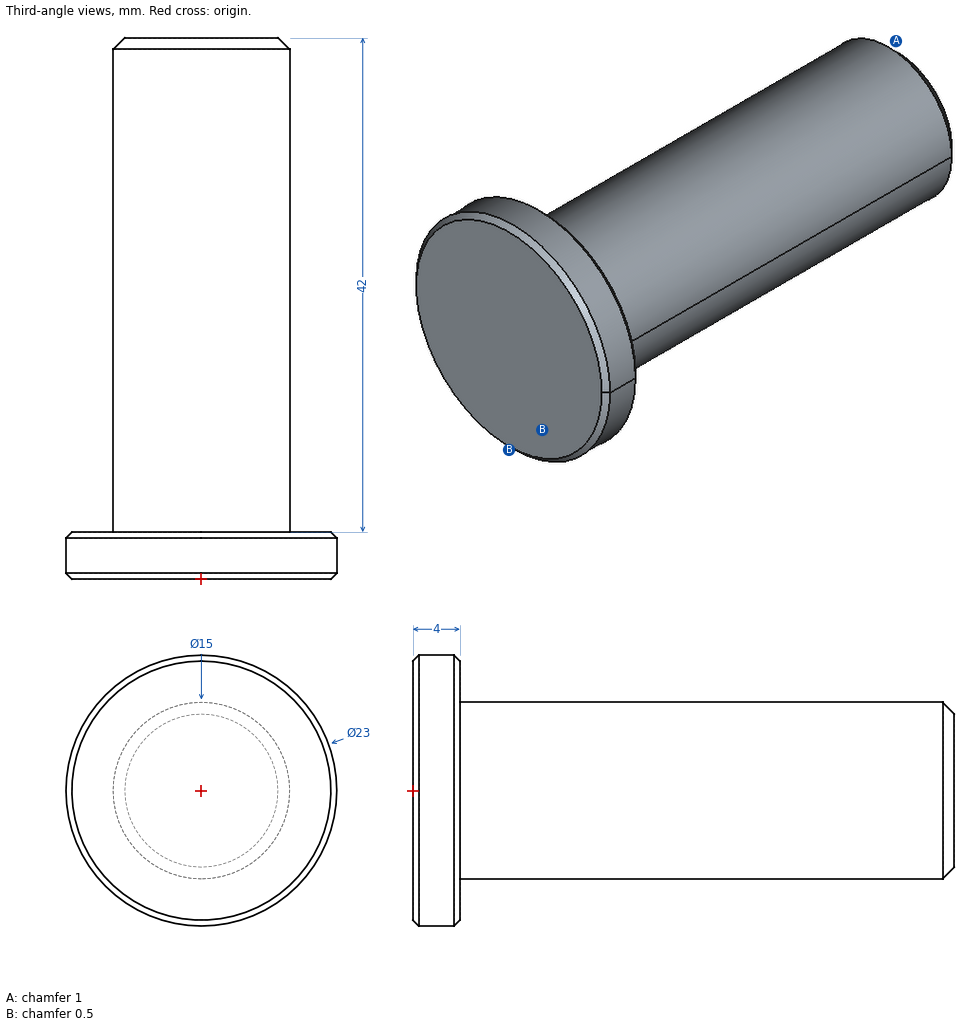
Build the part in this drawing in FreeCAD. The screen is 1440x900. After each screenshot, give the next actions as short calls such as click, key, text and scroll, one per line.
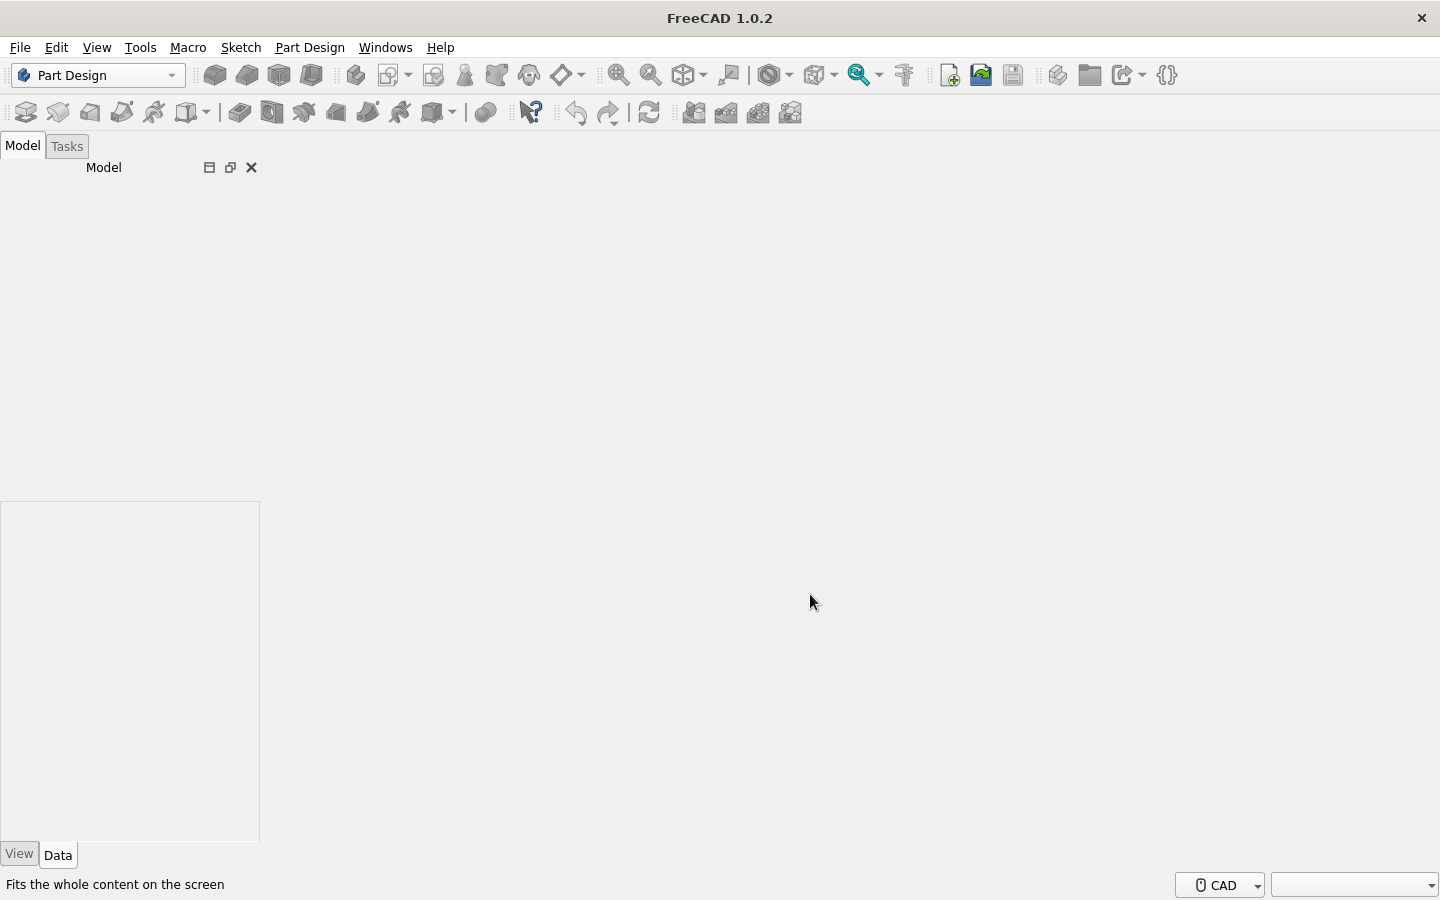
click(950, 76)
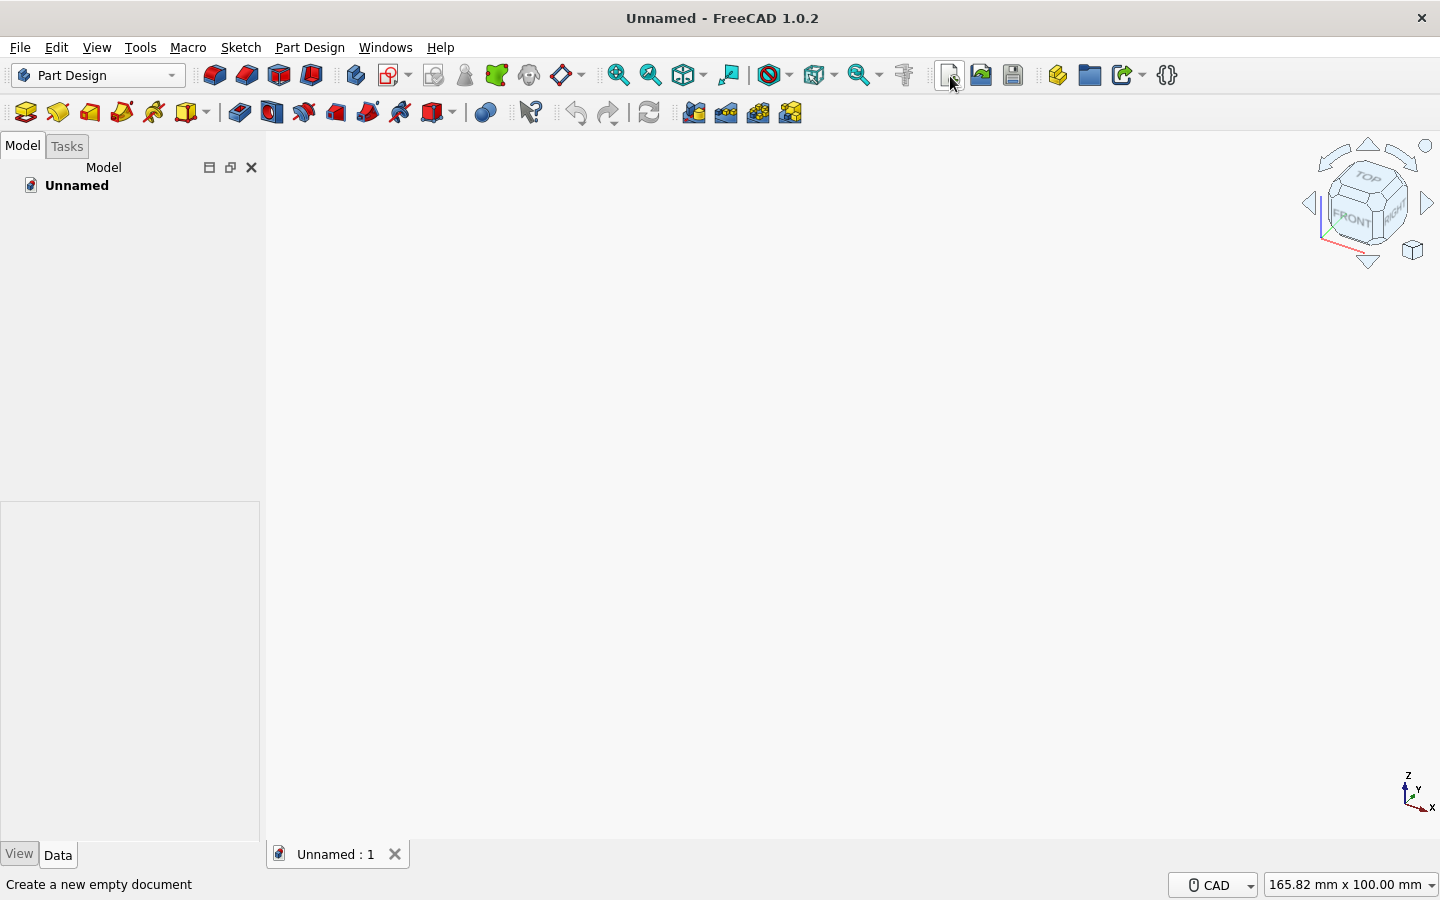
click(388, 76)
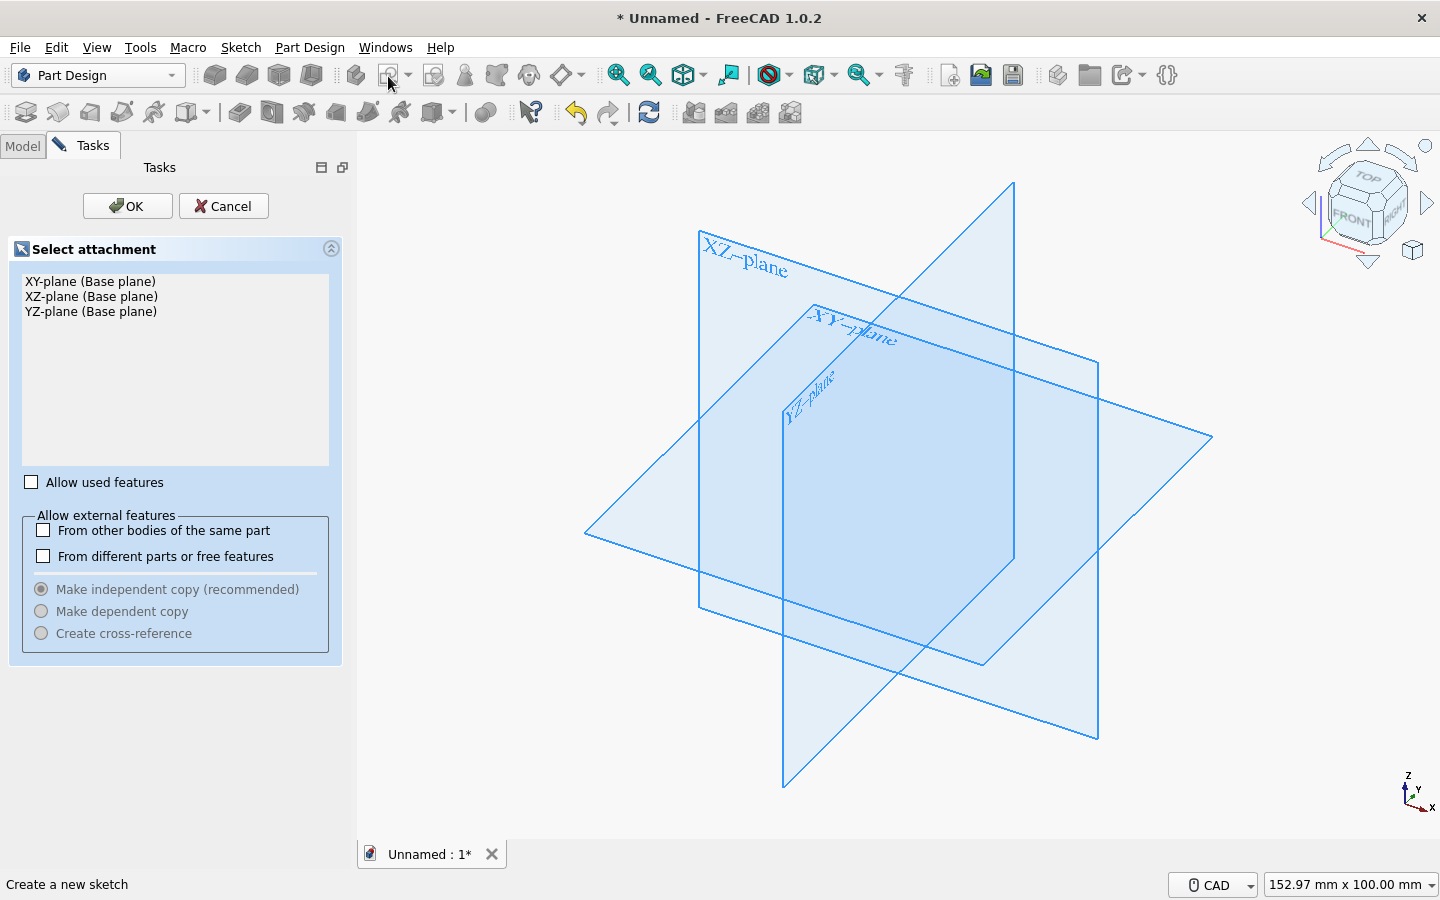
click(82, 296)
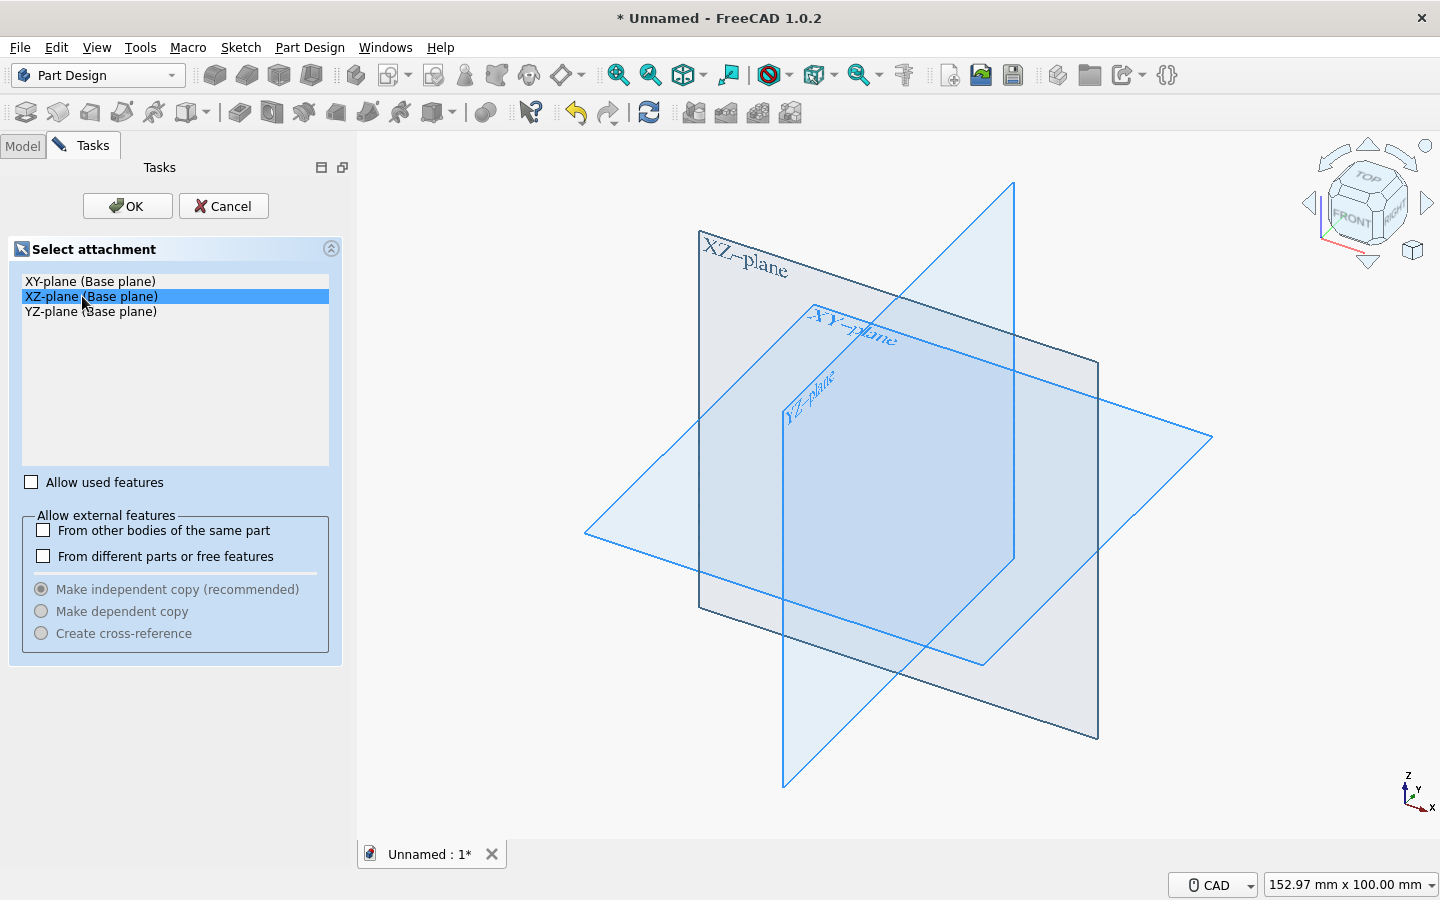
click(128, 206)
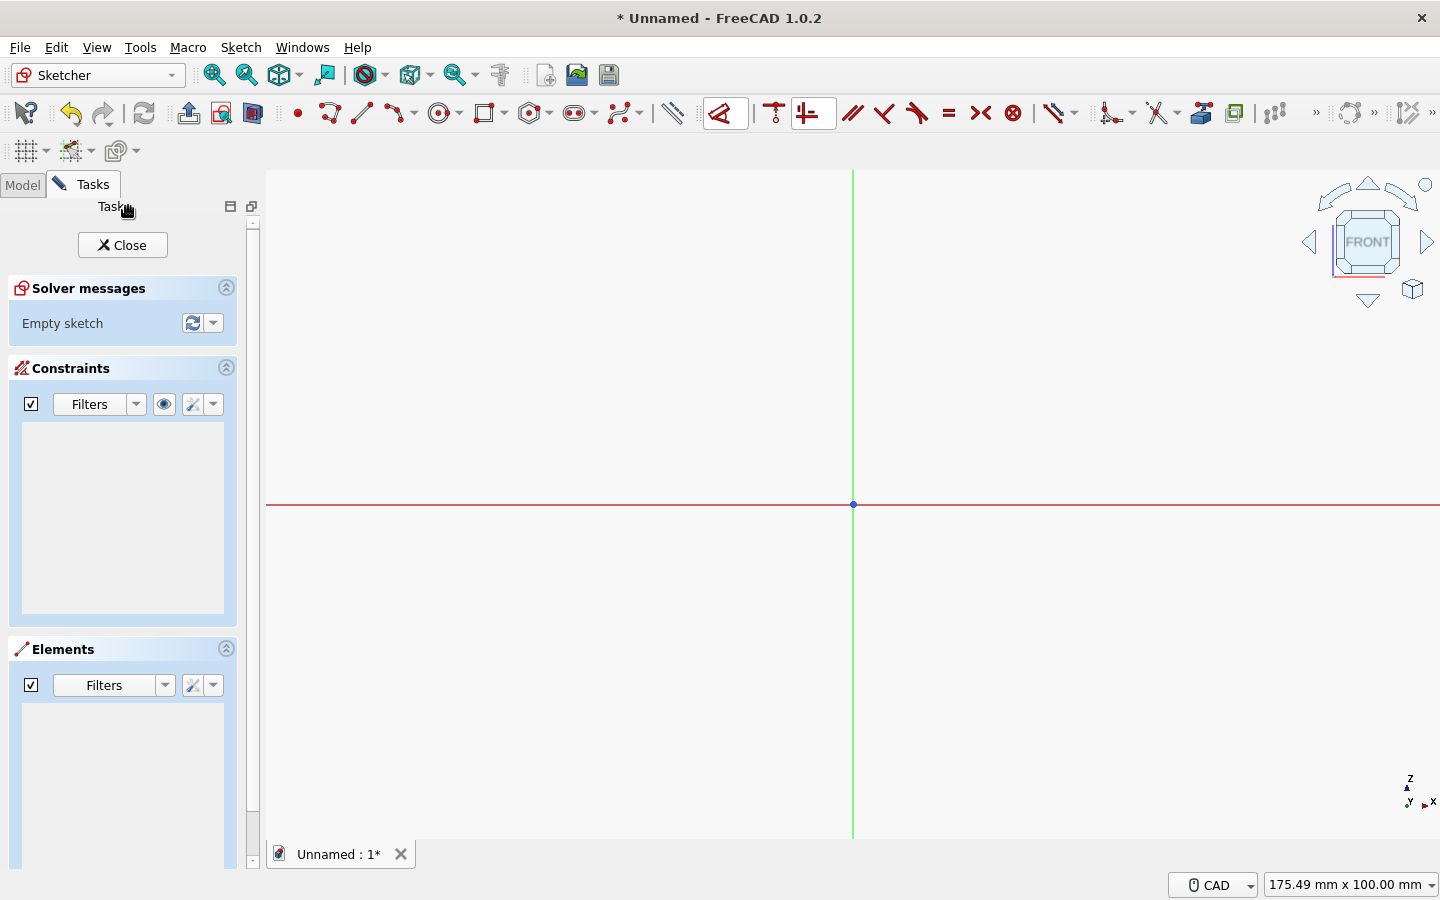
scroll(893, 504, up, 5)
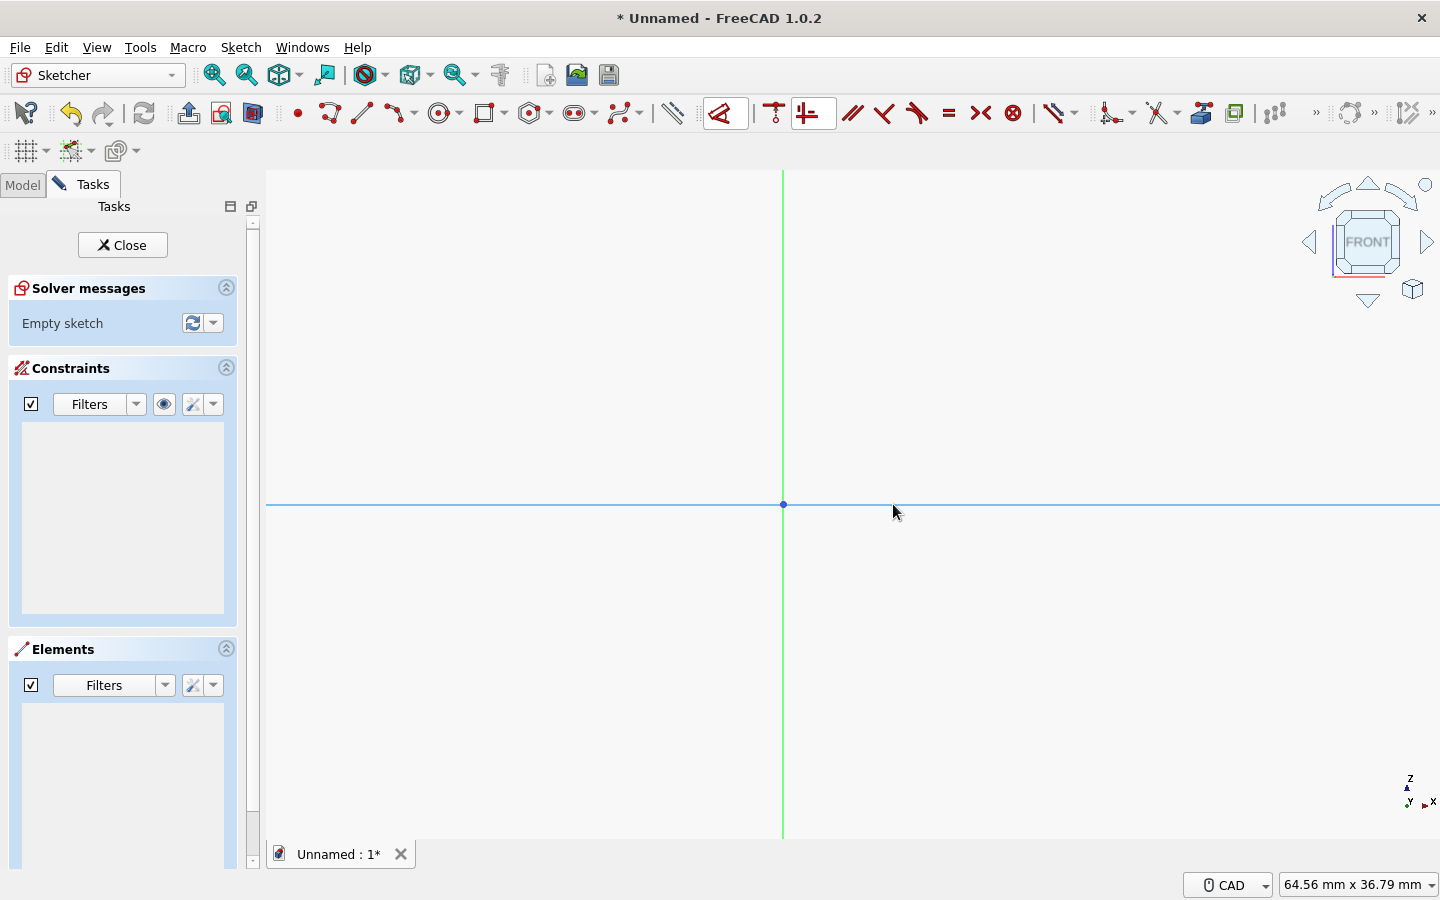
click(440, 114)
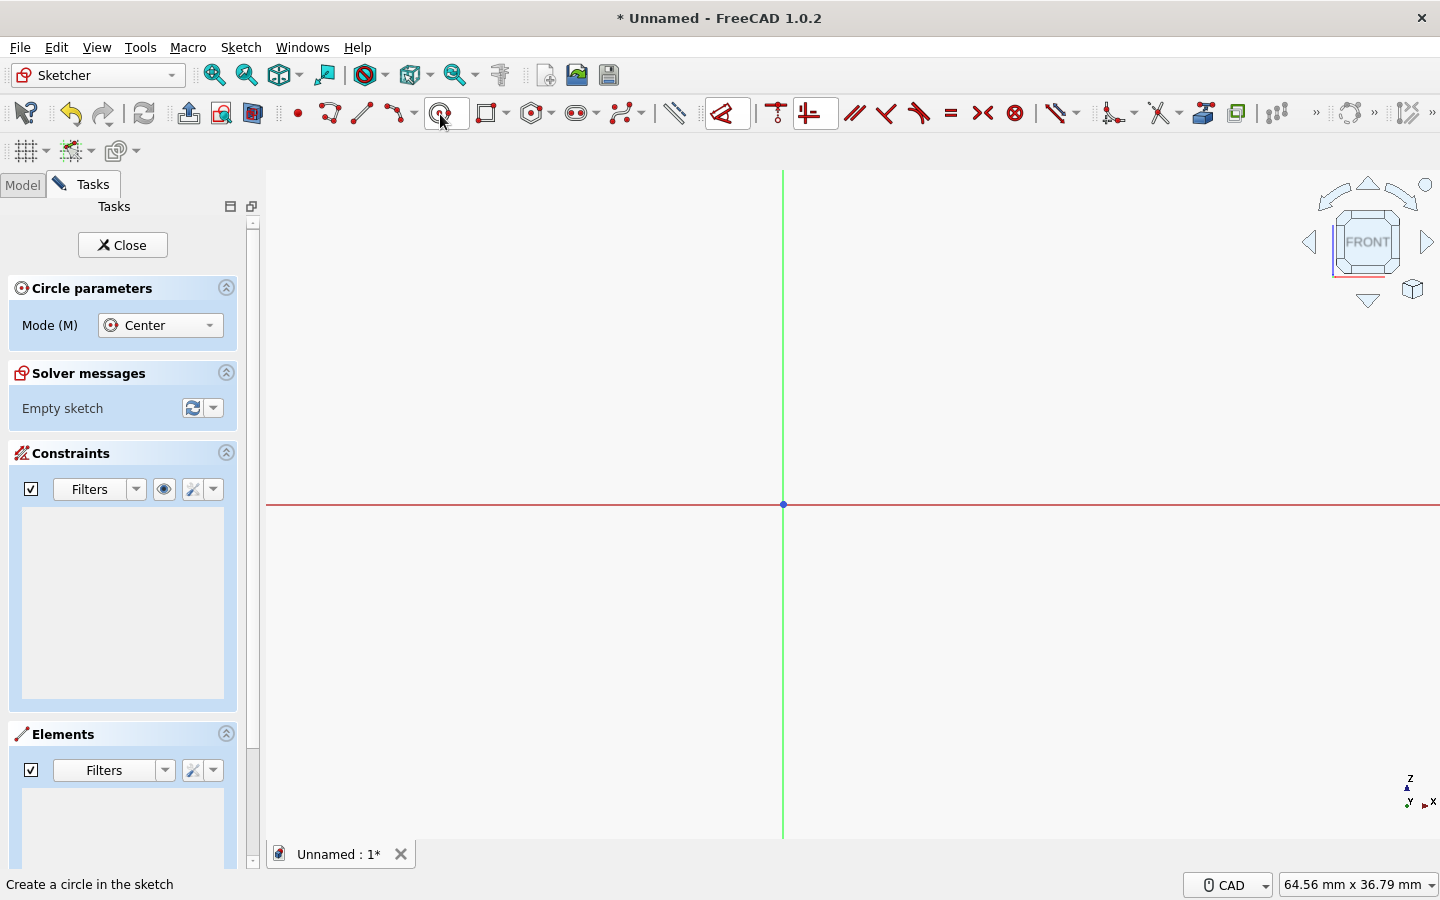
click(783, 504)
move(931, 357)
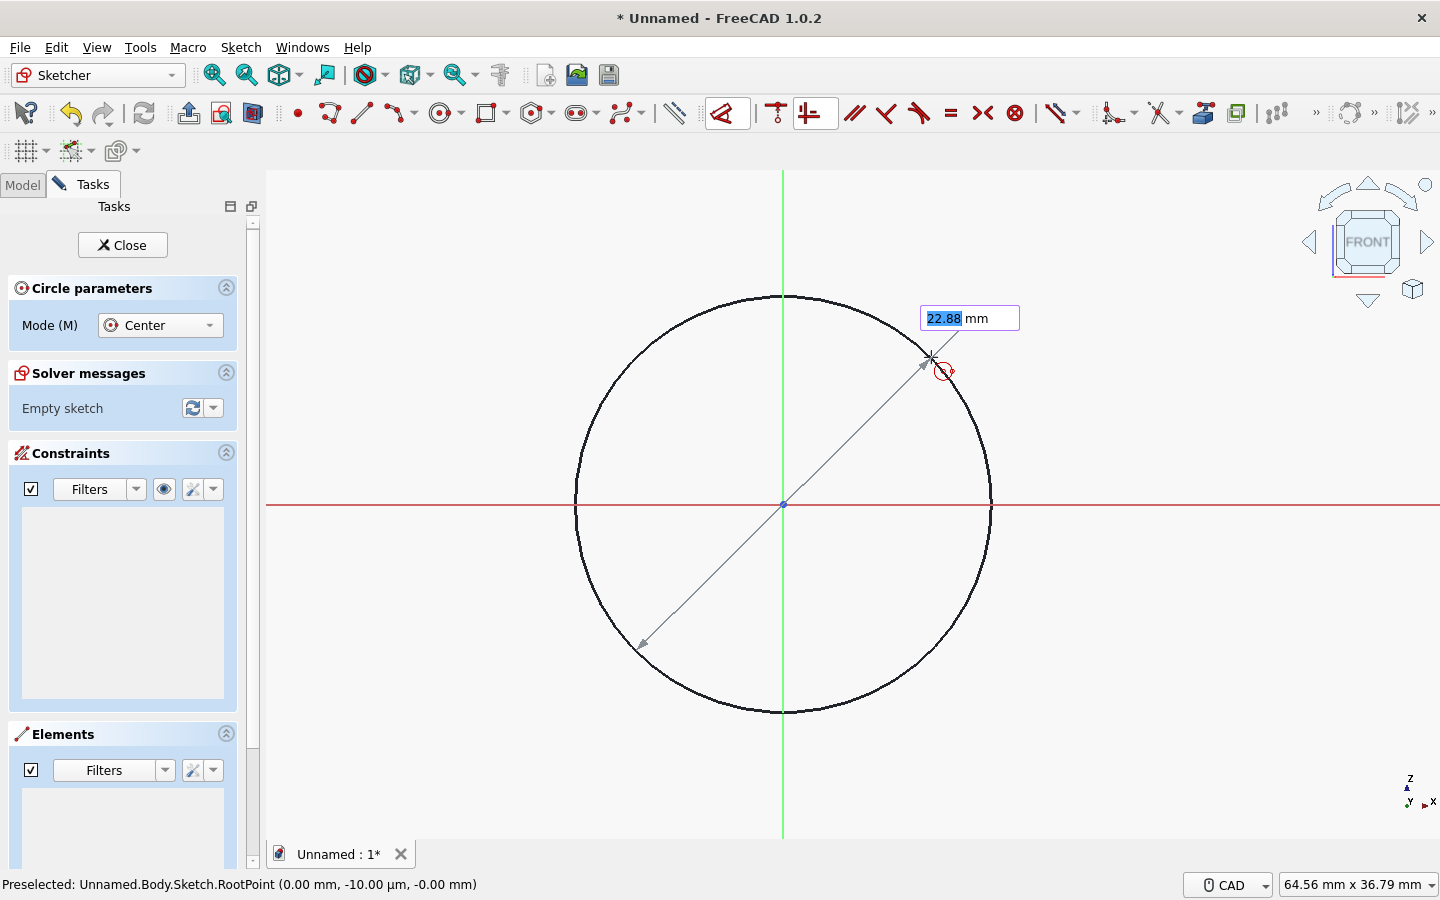
text(23)
key(Return)
key(Escape)